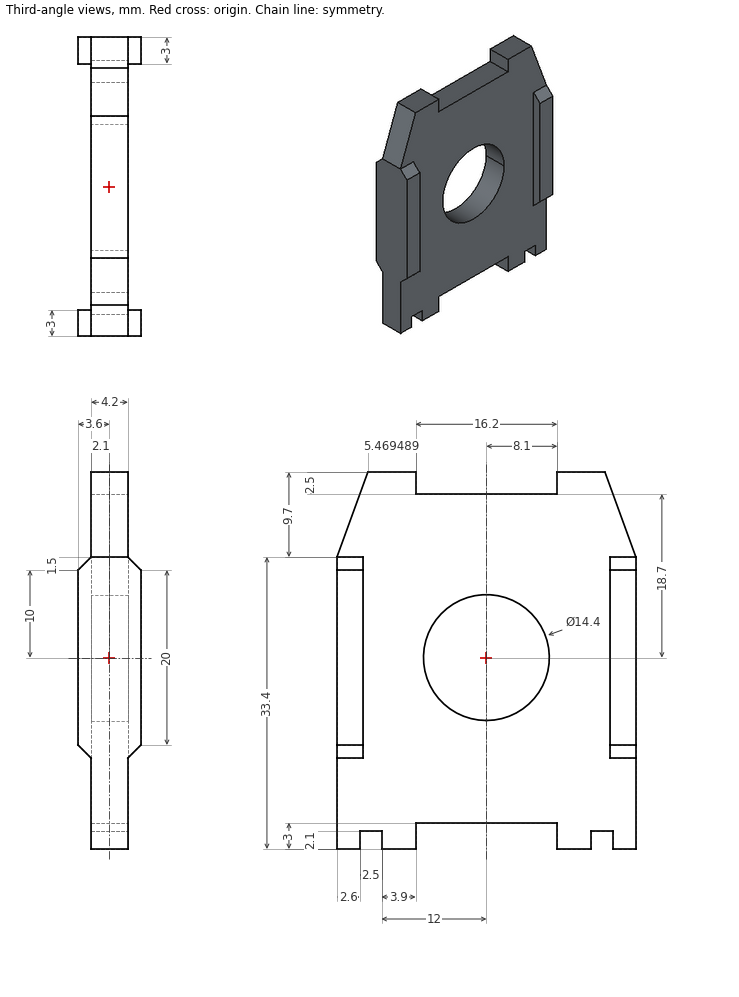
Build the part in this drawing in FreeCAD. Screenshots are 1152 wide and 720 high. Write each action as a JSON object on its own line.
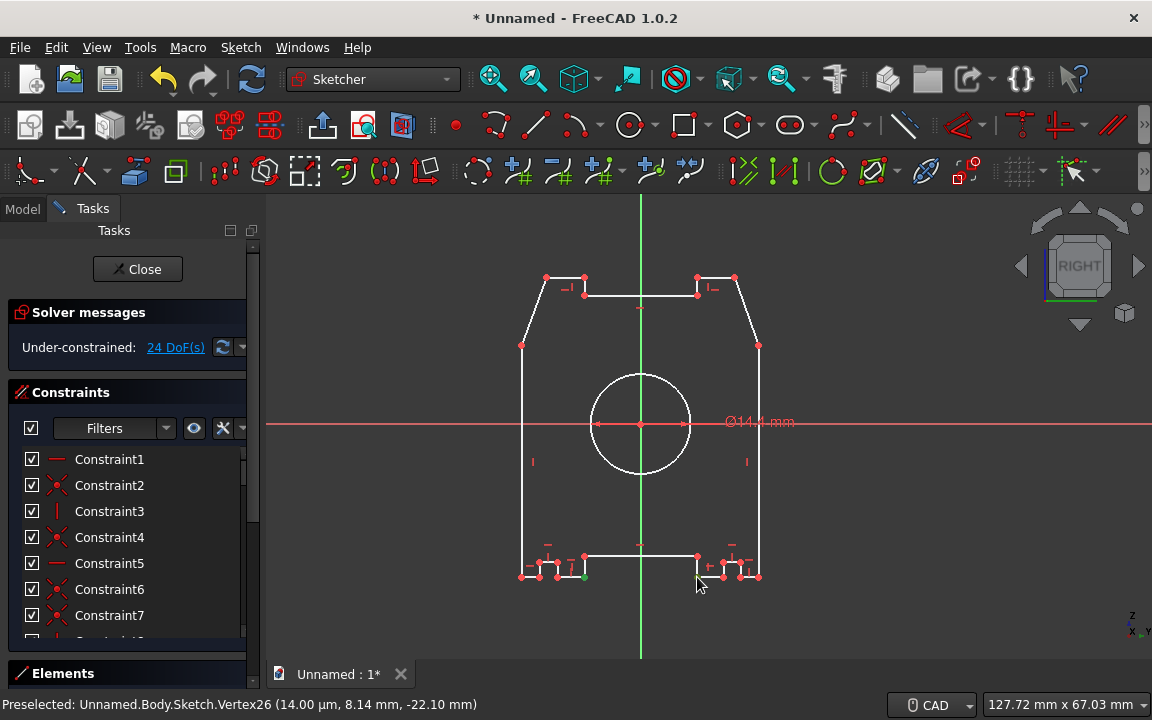
{"action": "left_click", "coordinate": [641, 602]}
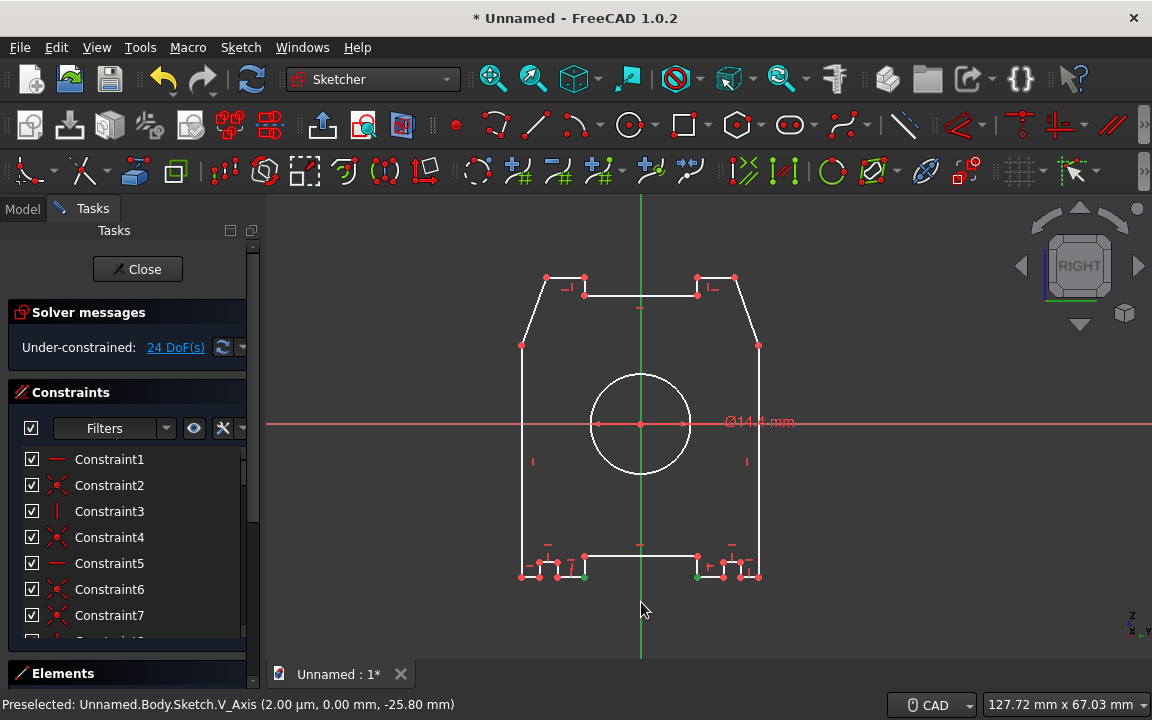
{"action": "key", "text": "s"}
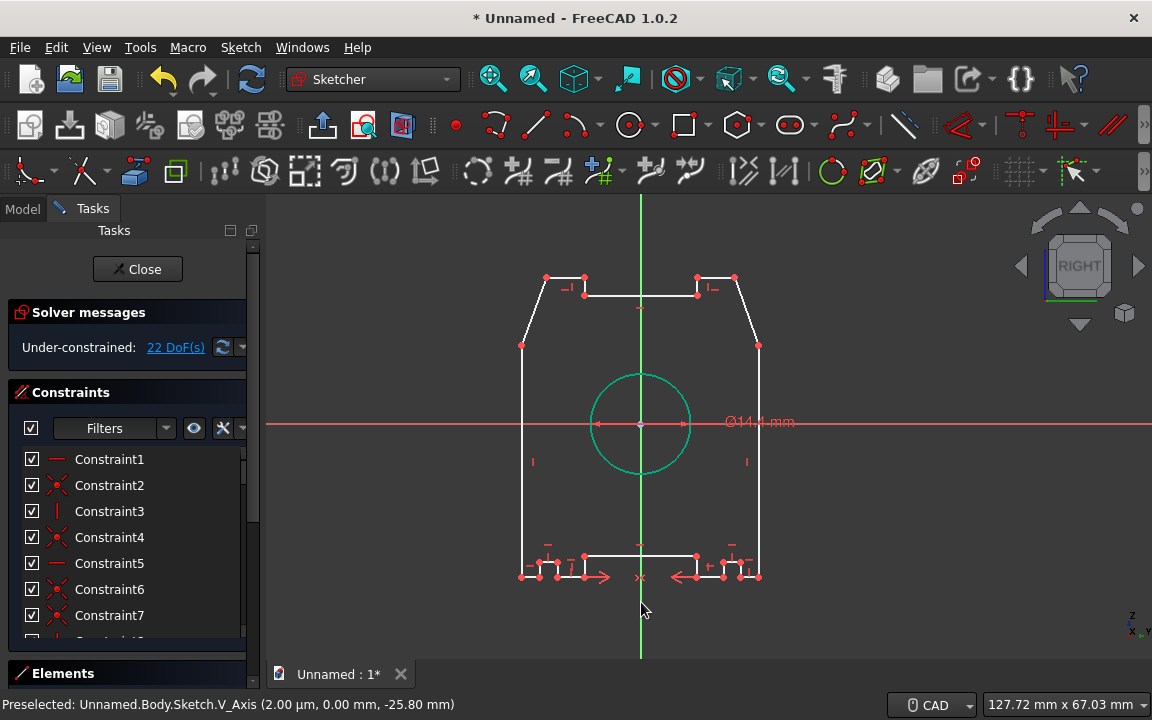
{"action": "left_click", "coordinate": [558, 562]}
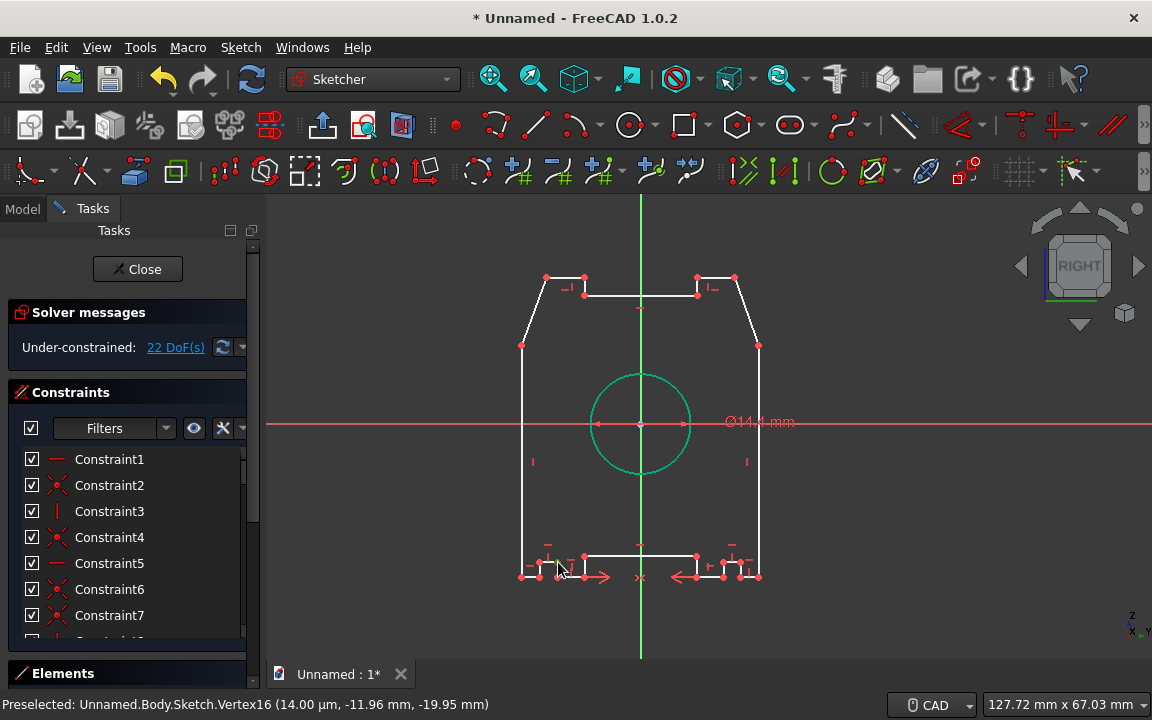
{"action": "left_click", "coordinate": [724, 562]}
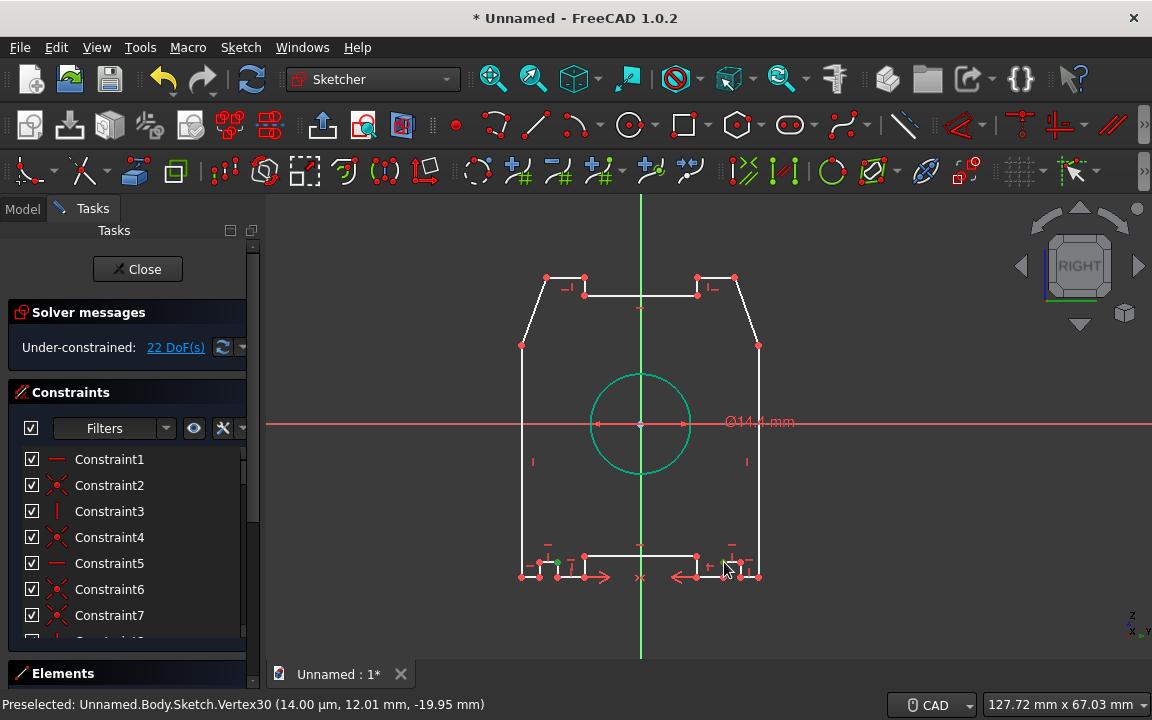
{"action": "left_click", "coordinate": [641, 602]}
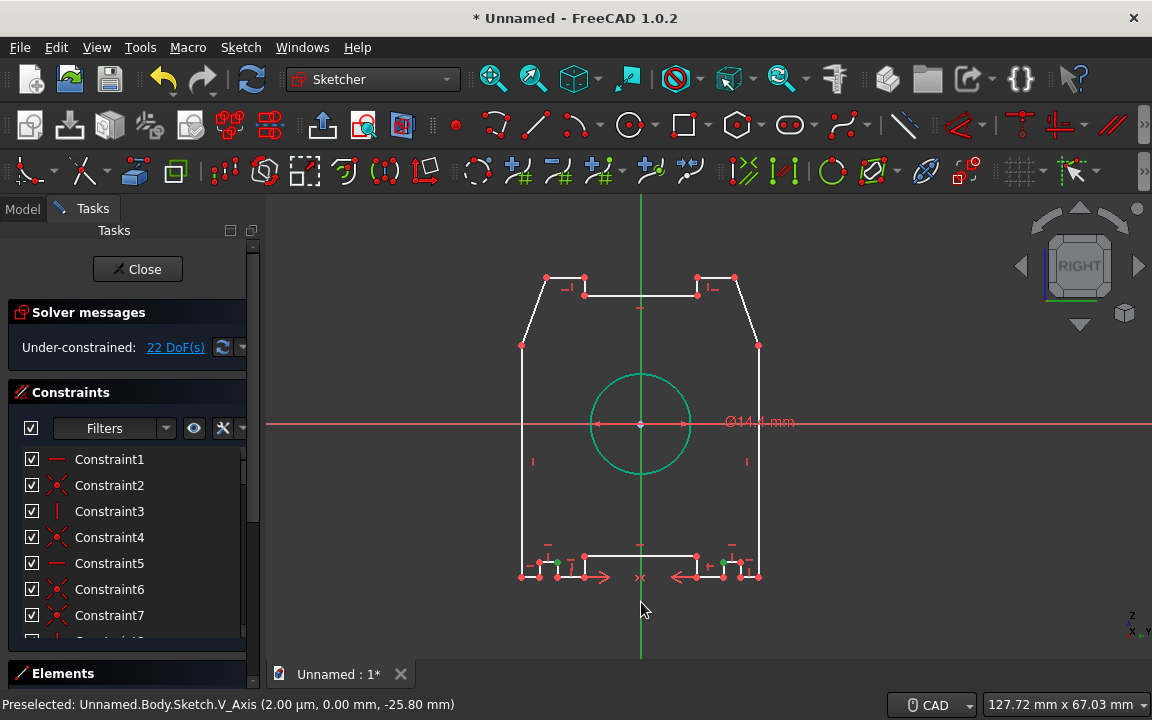
{"action": "key", "text": "s"}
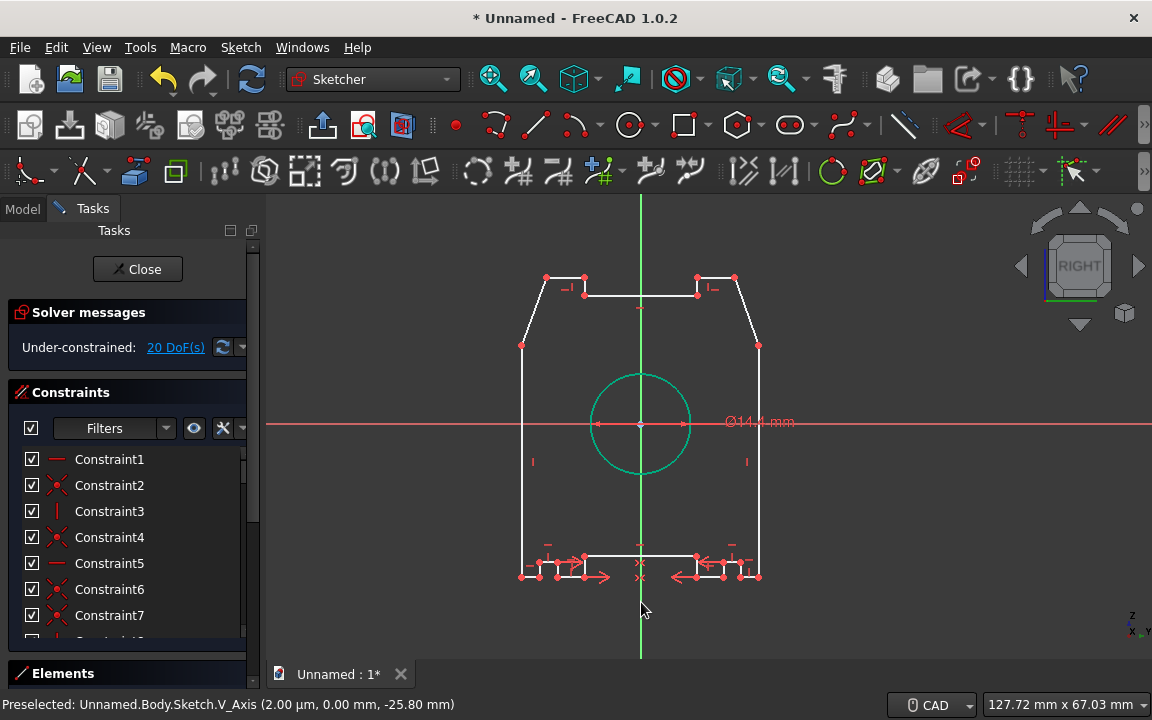
{"action": "left_click", "coordinate": [540, 577]}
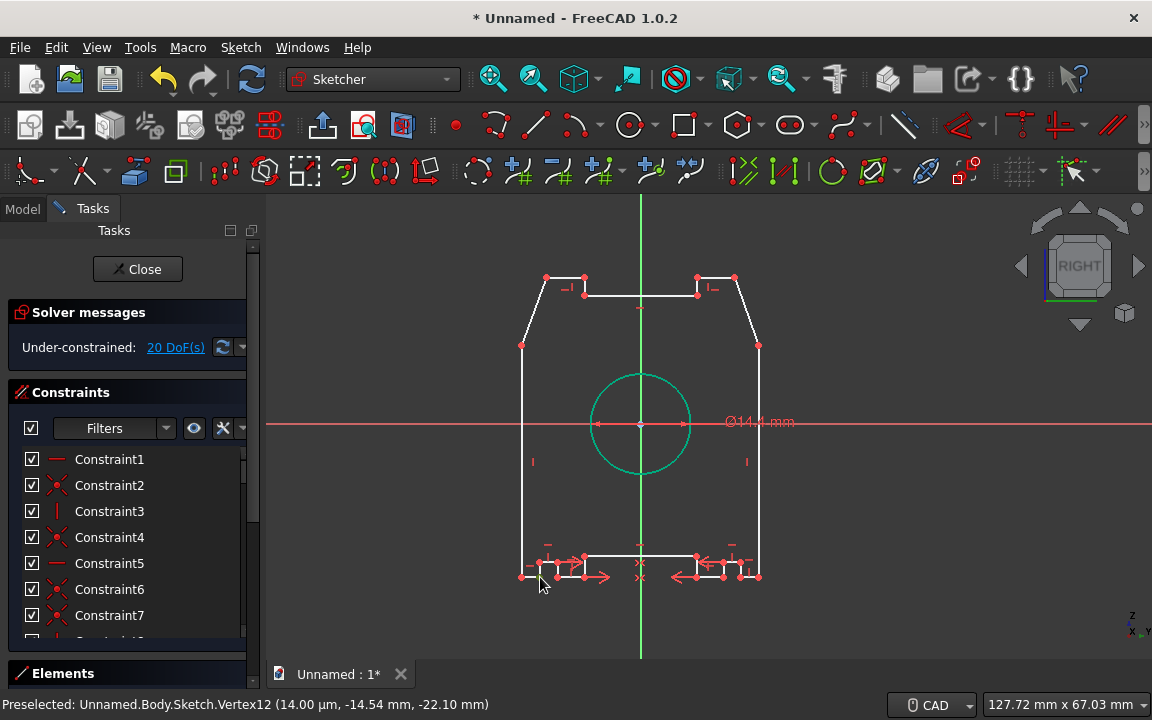
{"action": "left_click", "coordinate": [741, 577]}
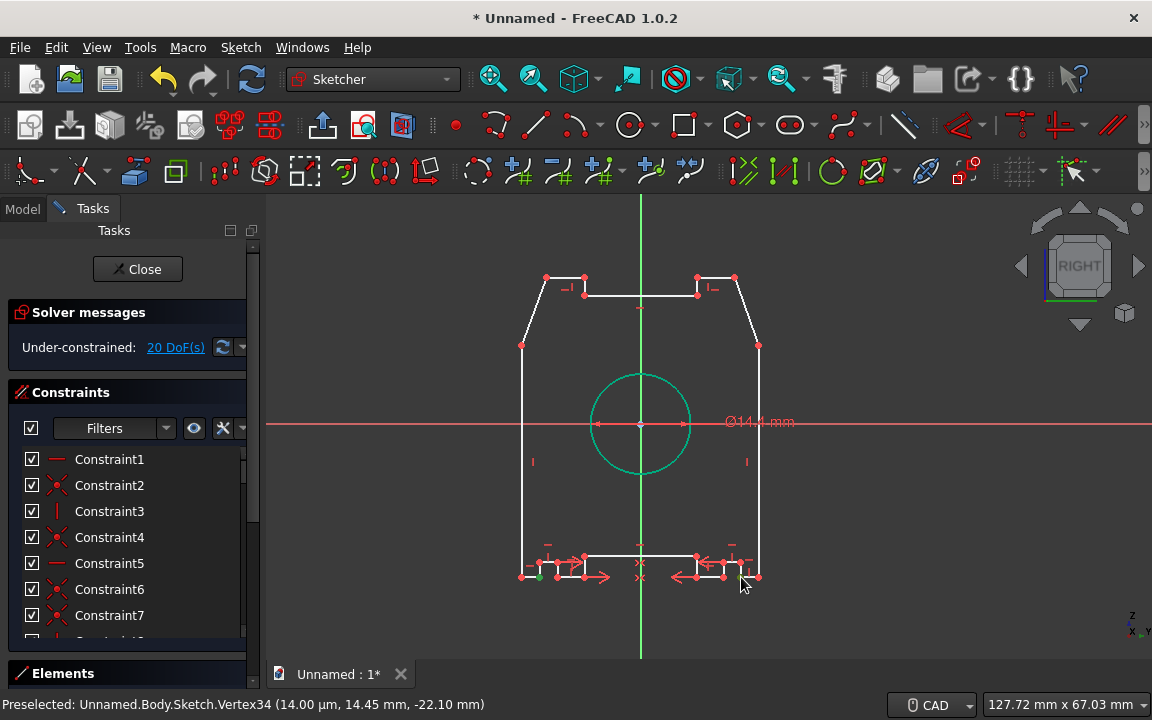
{"action": "left_click", "coordinate": [641, 602]}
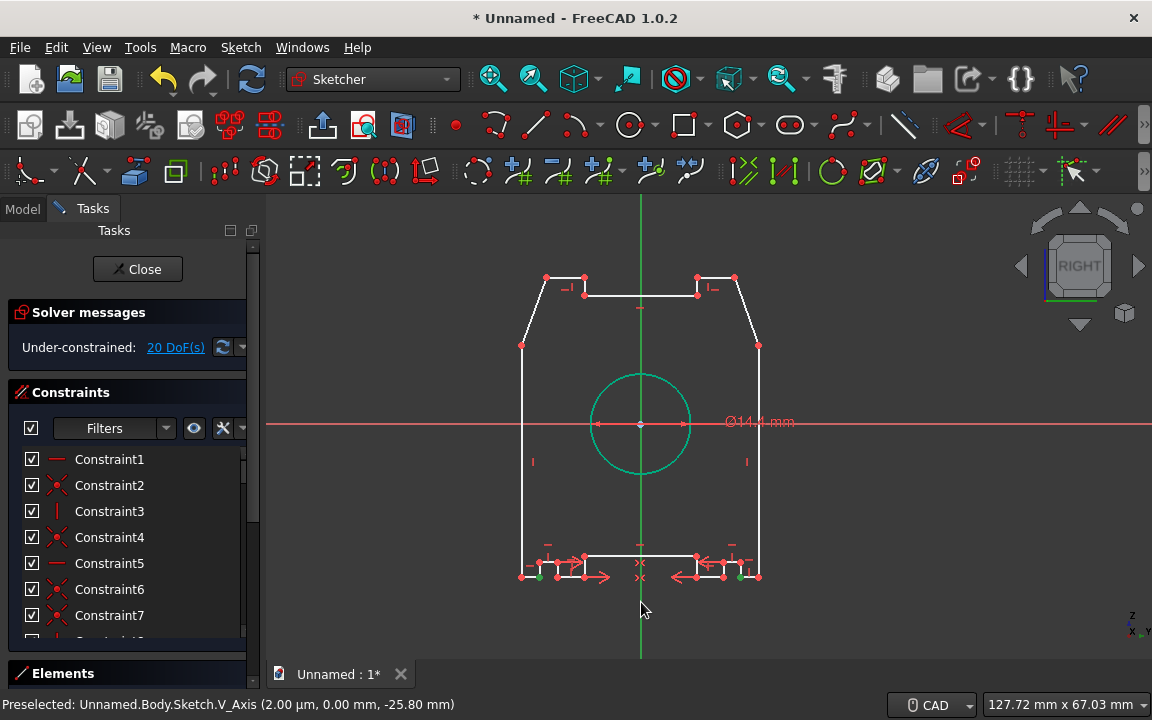
{"action": "key", "text": "s"}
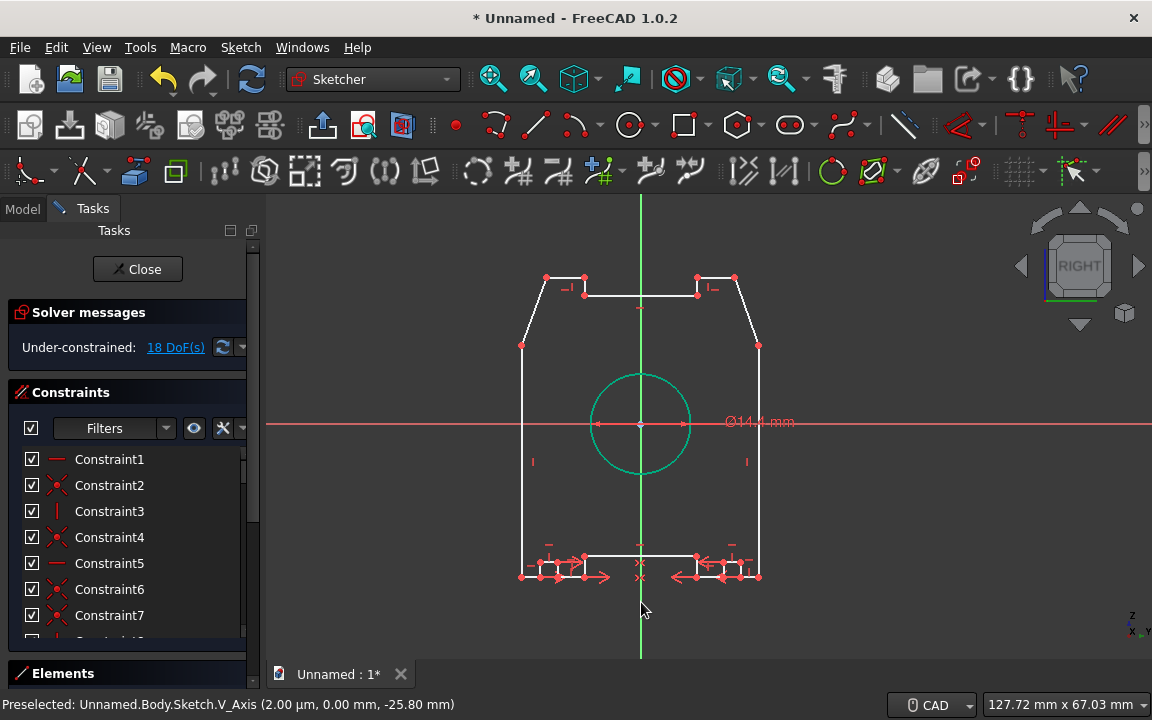
{"action": "left_click", "coordinate": [522, 345]}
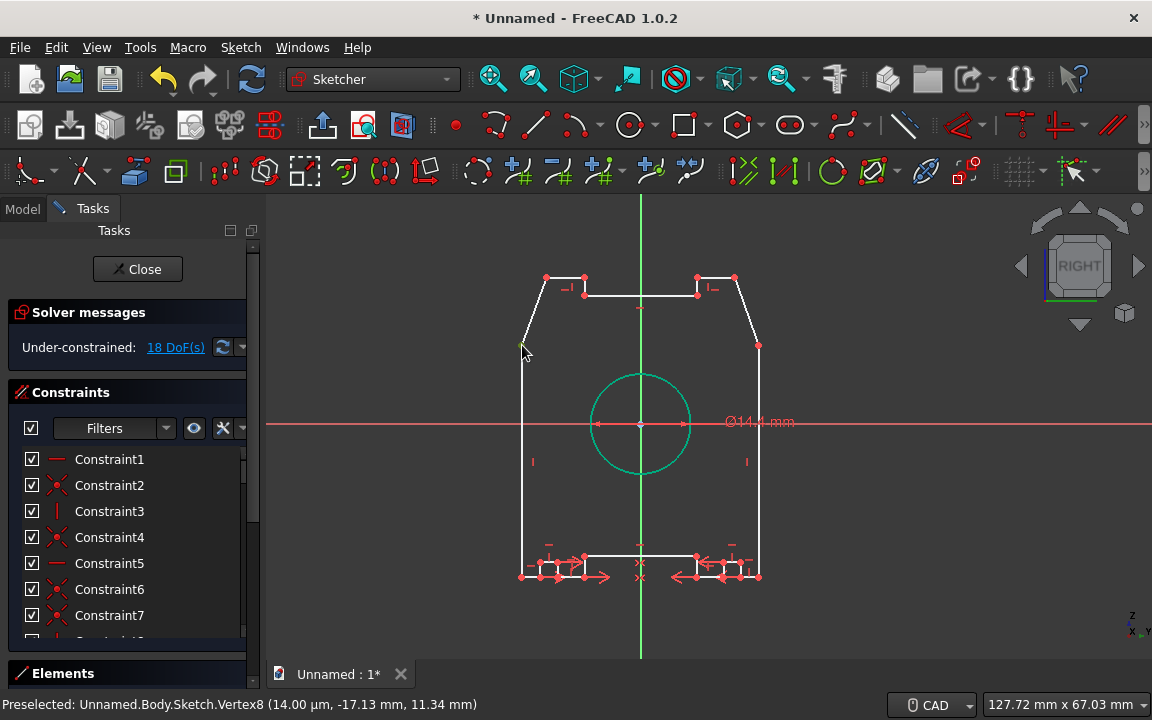
{"action": "left_click", "coordinate": [759, 345]}